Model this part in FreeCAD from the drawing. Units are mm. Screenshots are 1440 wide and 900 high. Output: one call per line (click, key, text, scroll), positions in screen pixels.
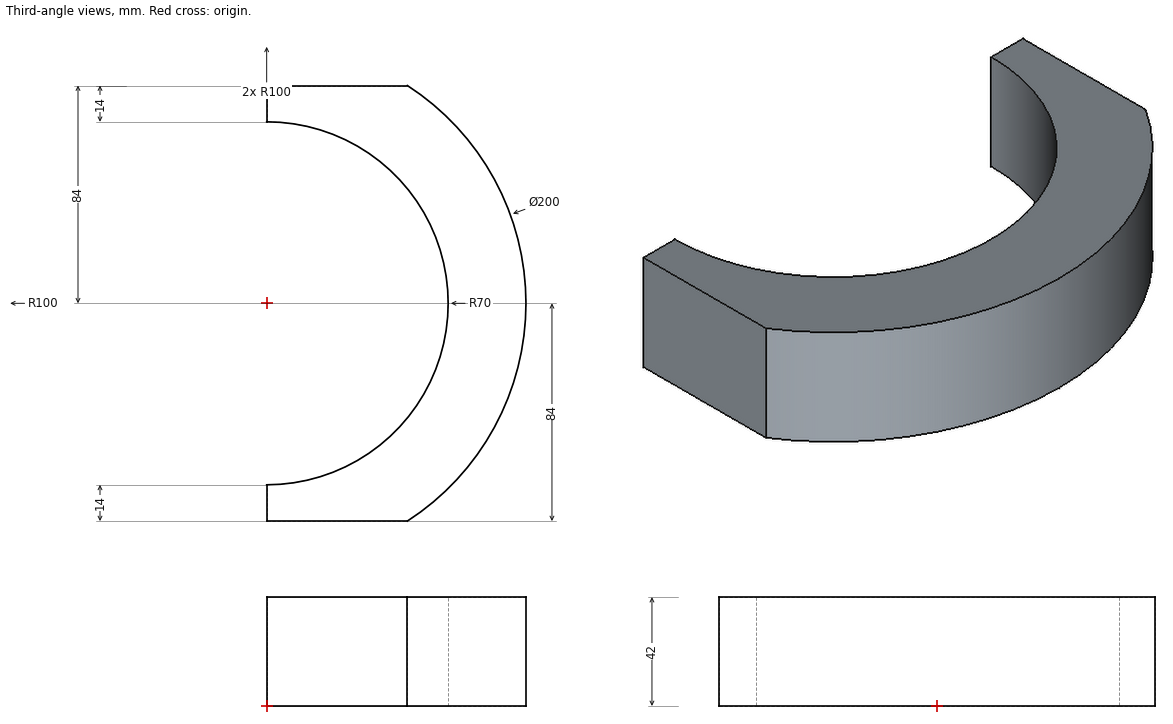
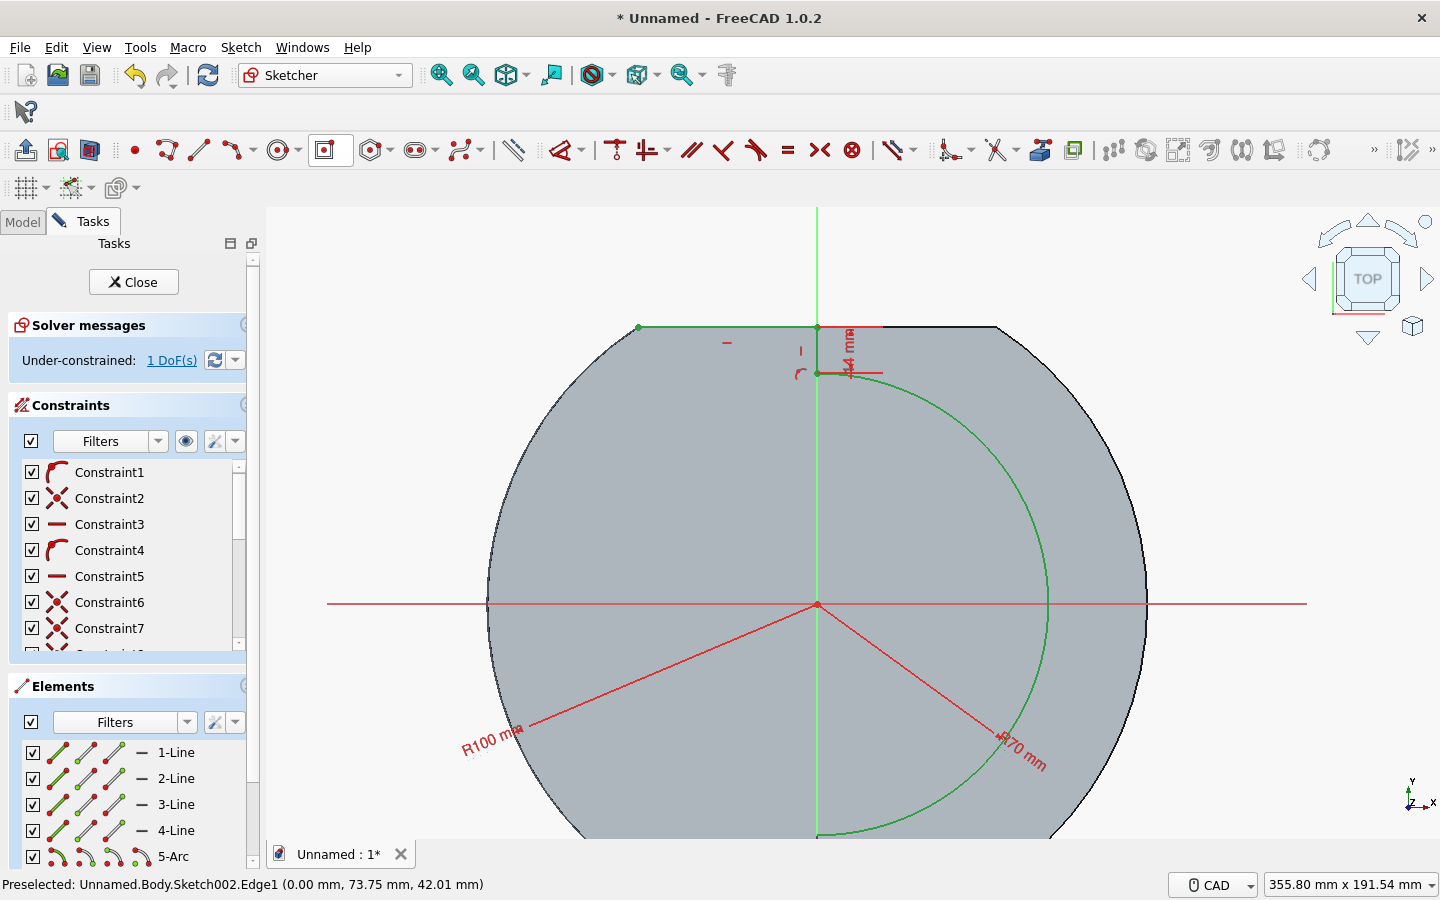
scroll(818, 358, down, 2)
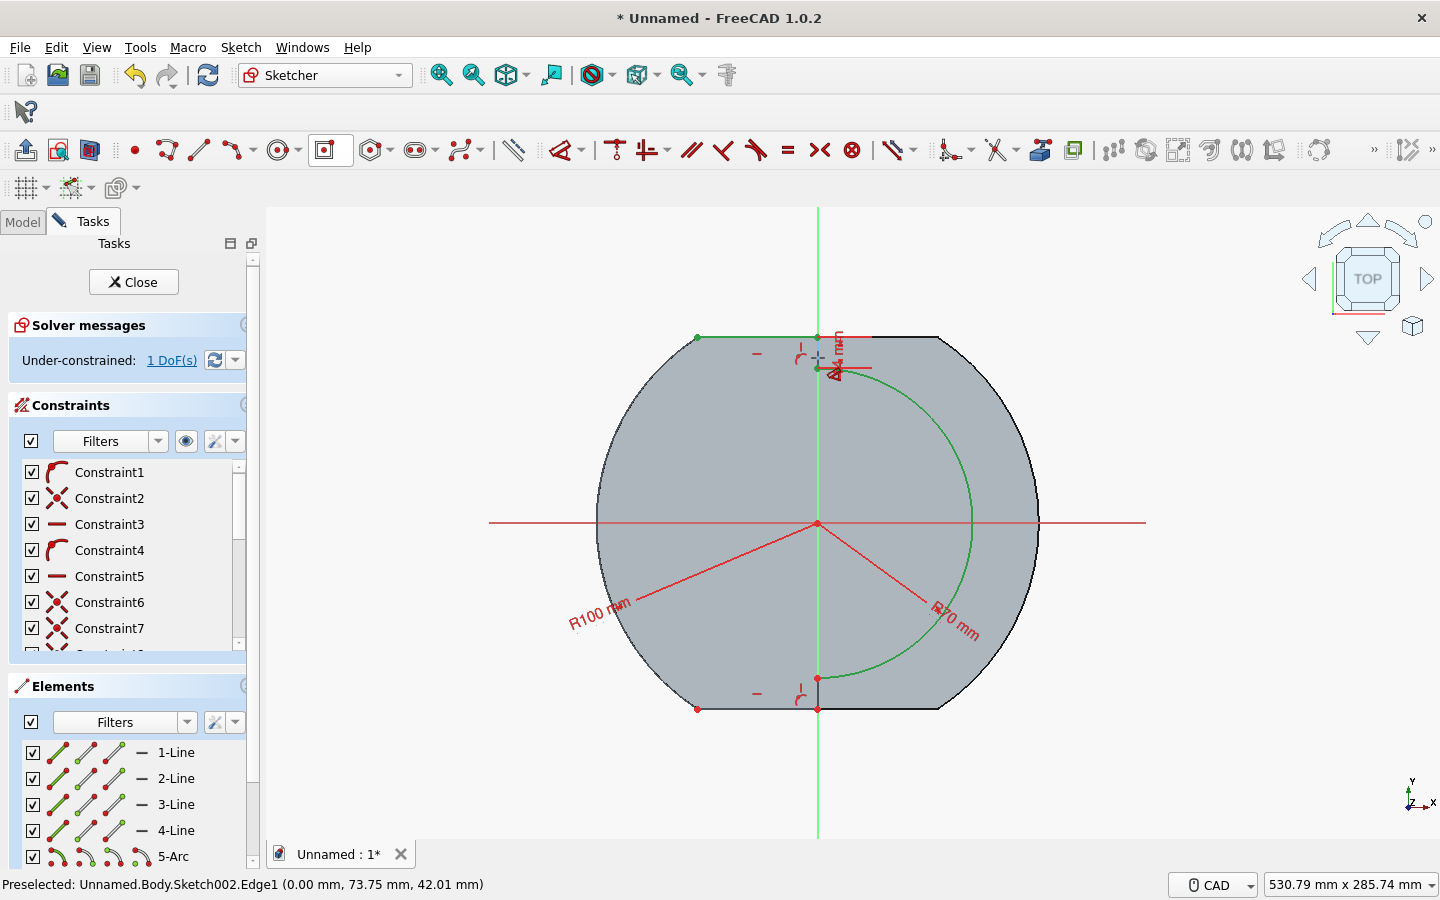
scroll(818, 700, up, 2)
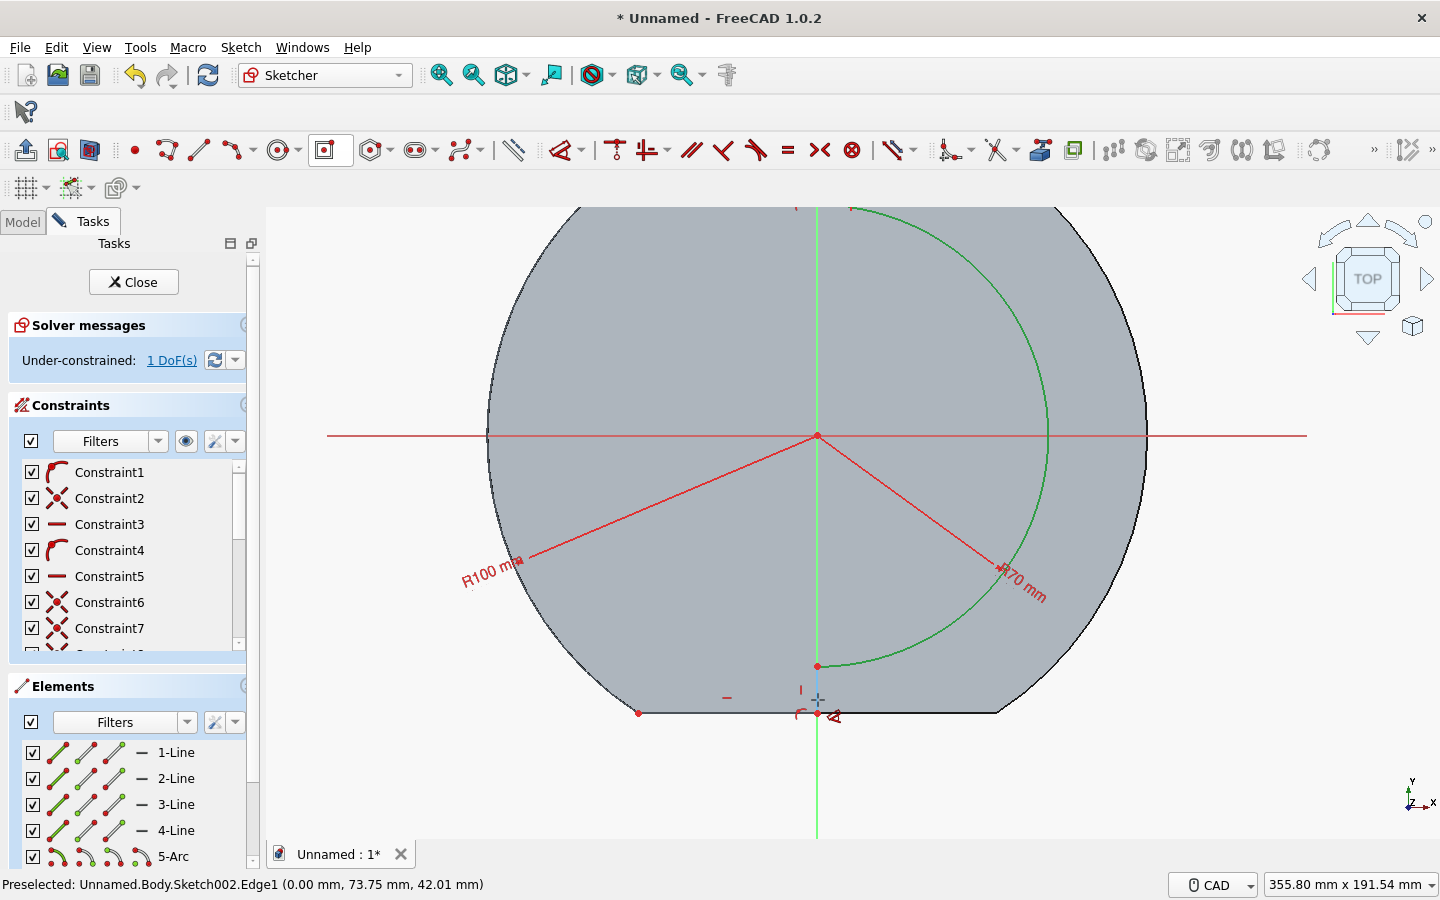
click(817, 699)
click(851, 690)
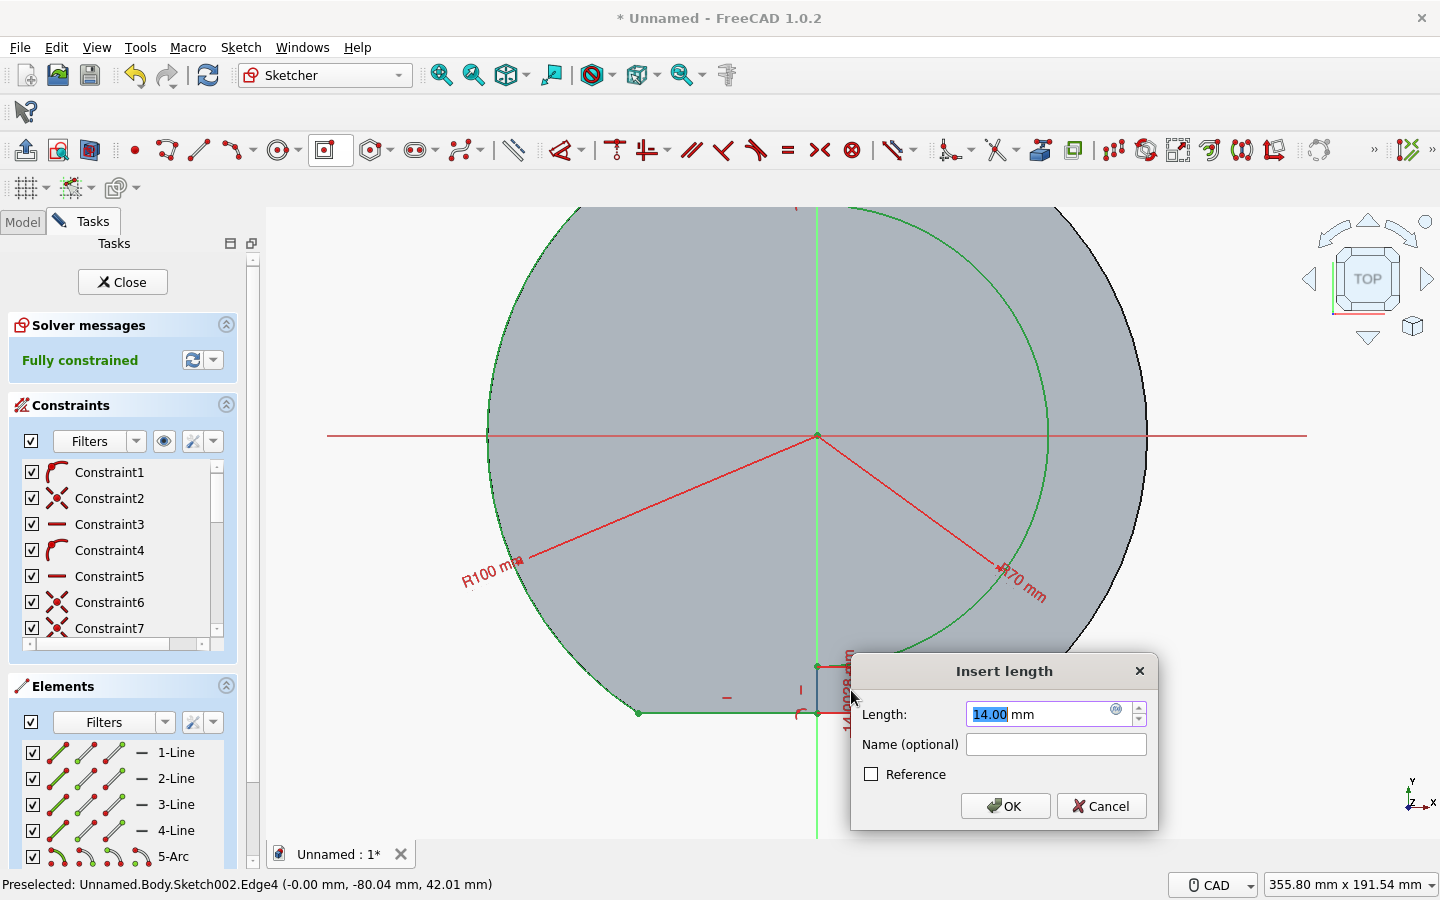
text(14)
key(Return)
key(Escape)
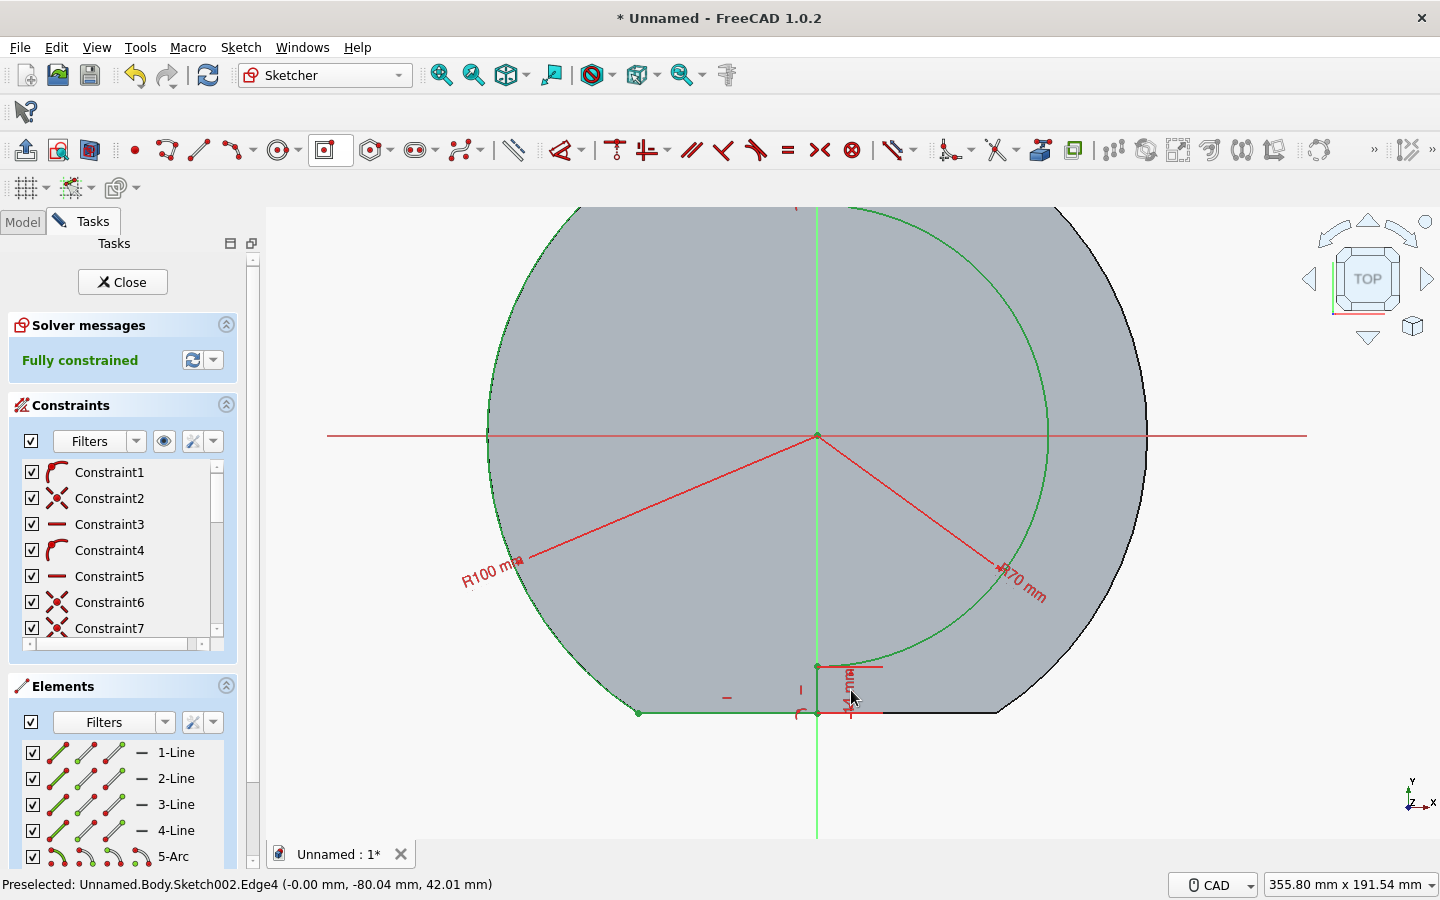
click(123, 282)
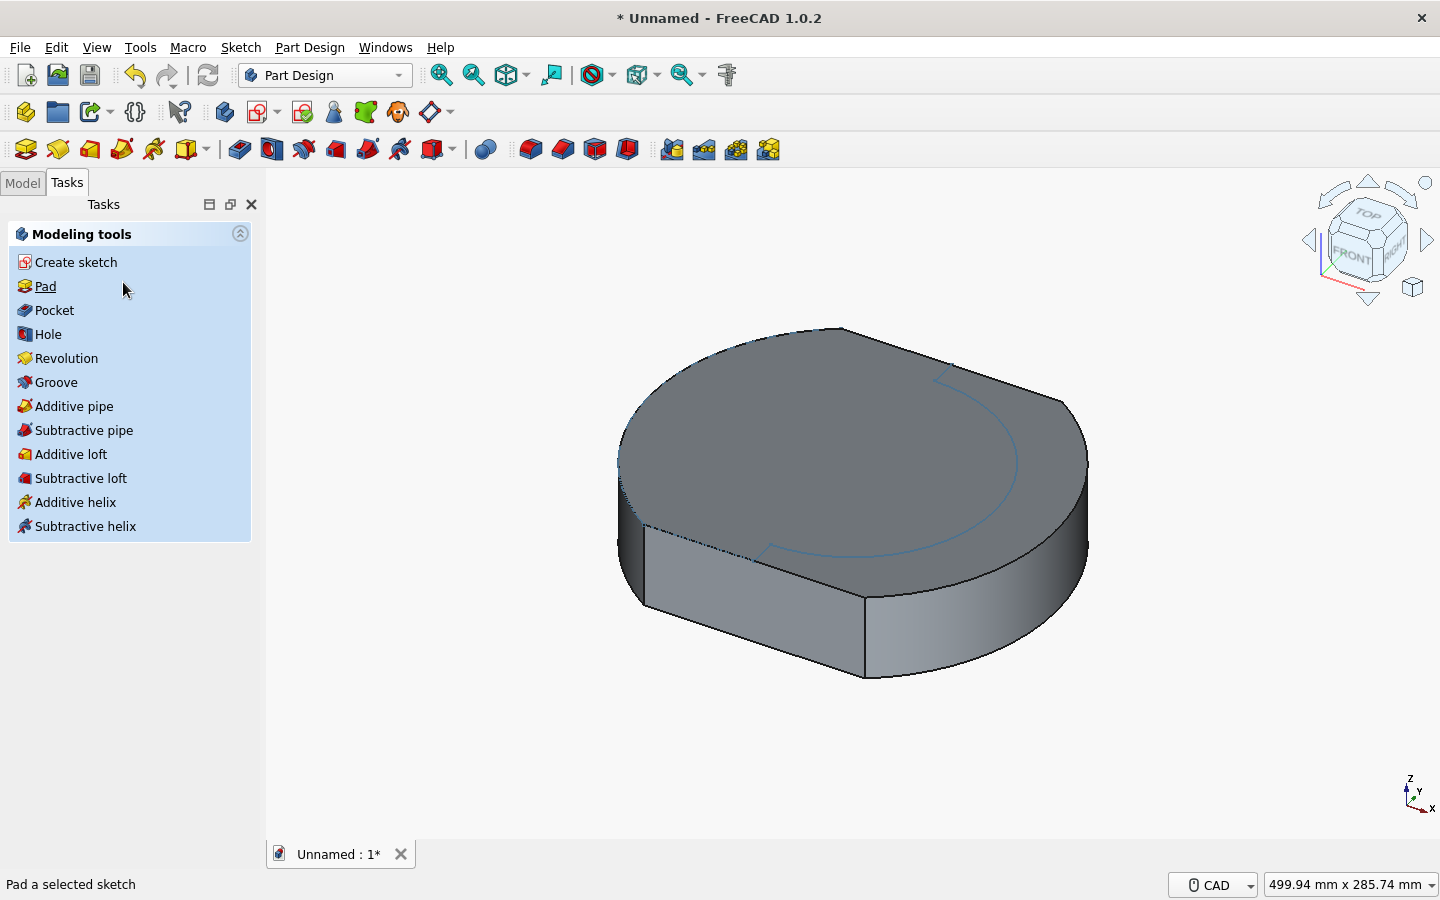
click(240, 150)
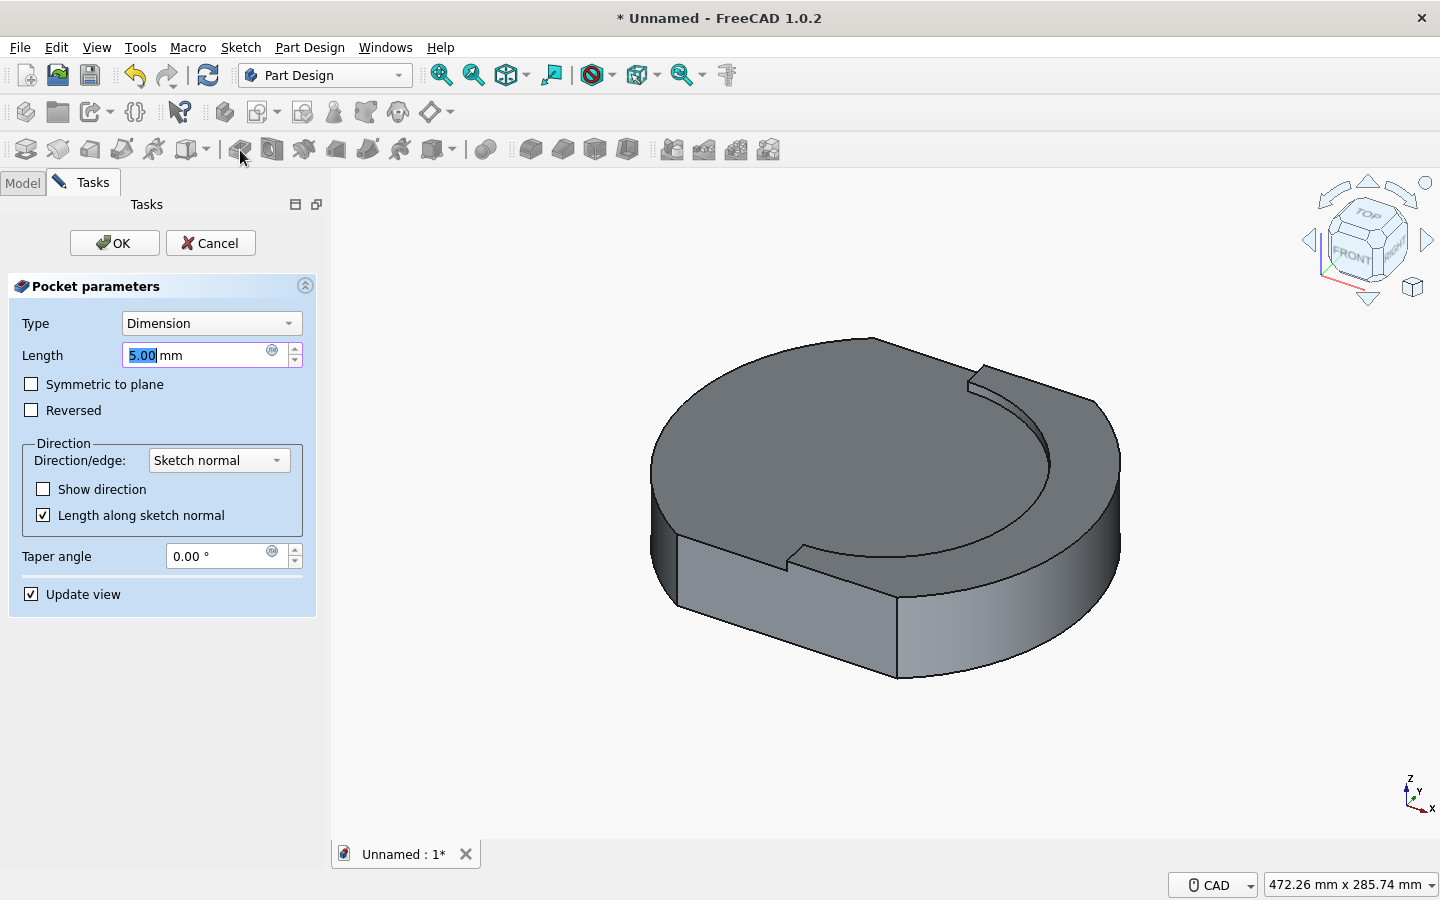
click(212, 324)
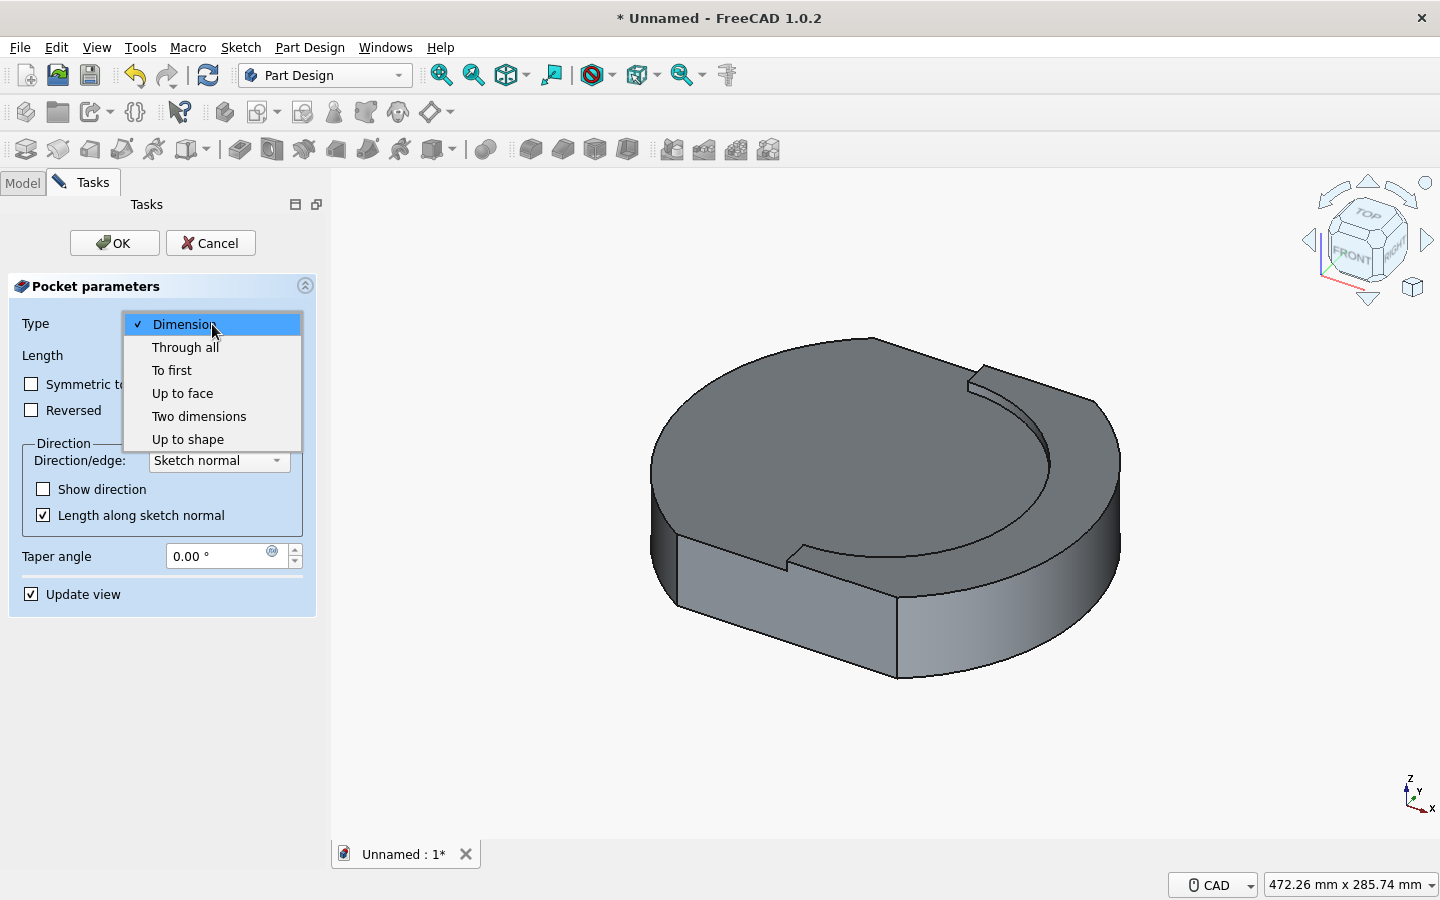
click(212, 348)